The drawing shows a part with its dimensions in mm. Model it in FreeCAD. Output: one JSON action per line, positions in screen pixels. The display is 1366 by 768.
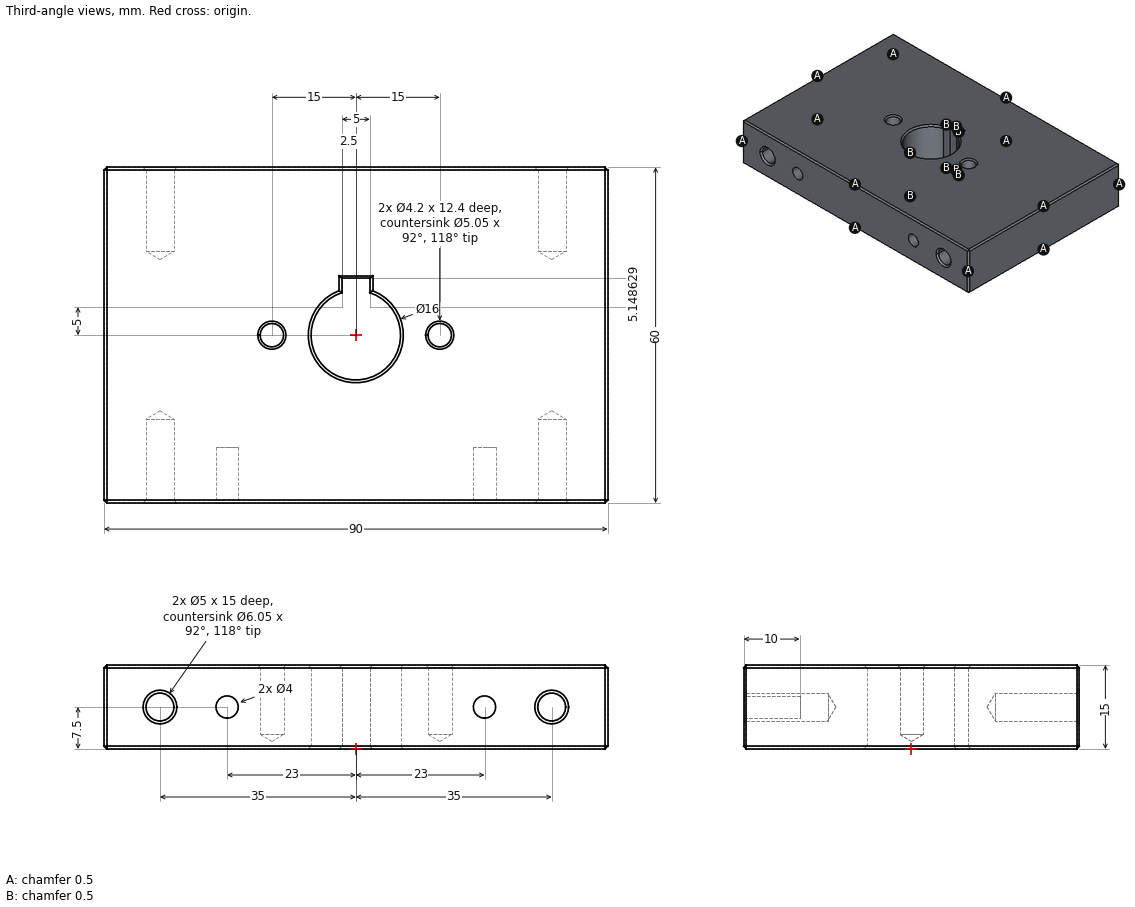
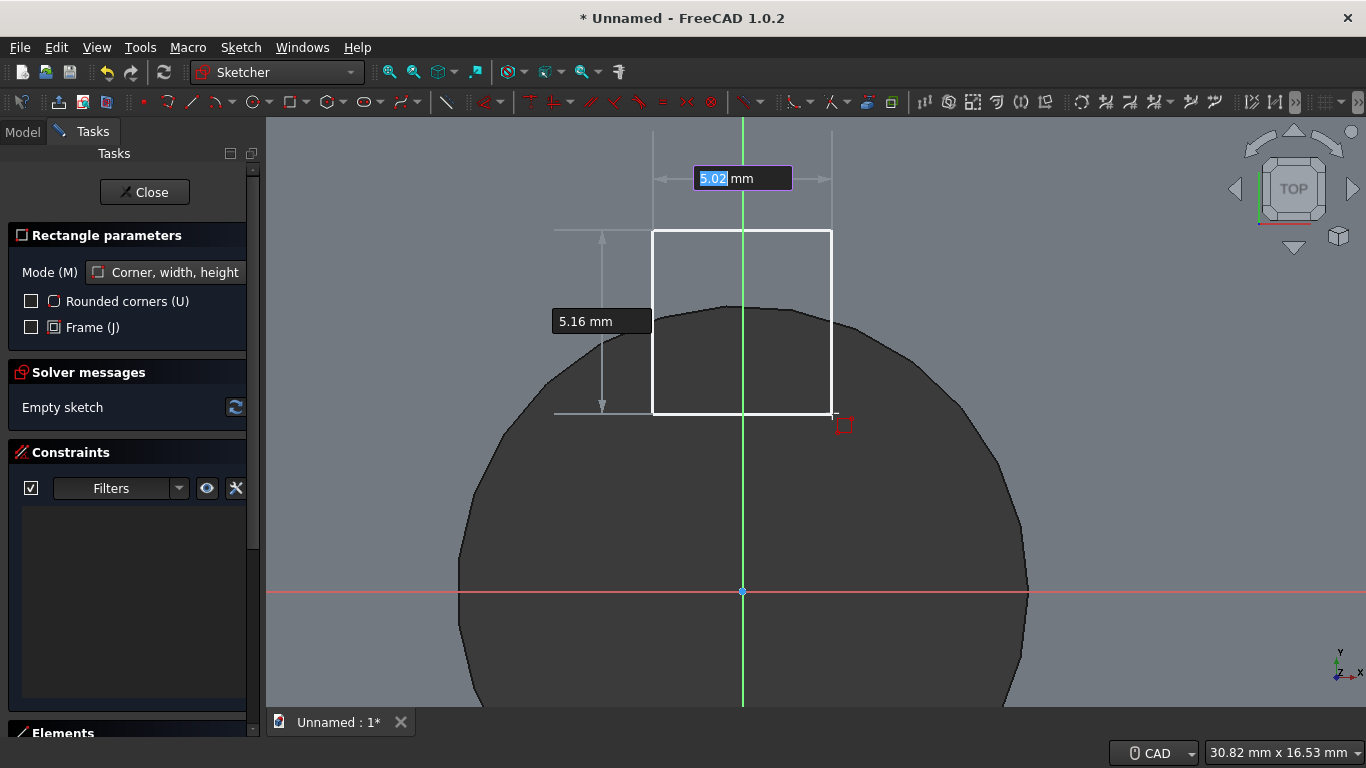
{"action": "type", "text": "5"}
{"action": "key", "text": "Tab"}
{"action": "type", "text": "5.148629"}
{"action": "key", "text": "Return"}
{"action": "key", "text": "Escape"}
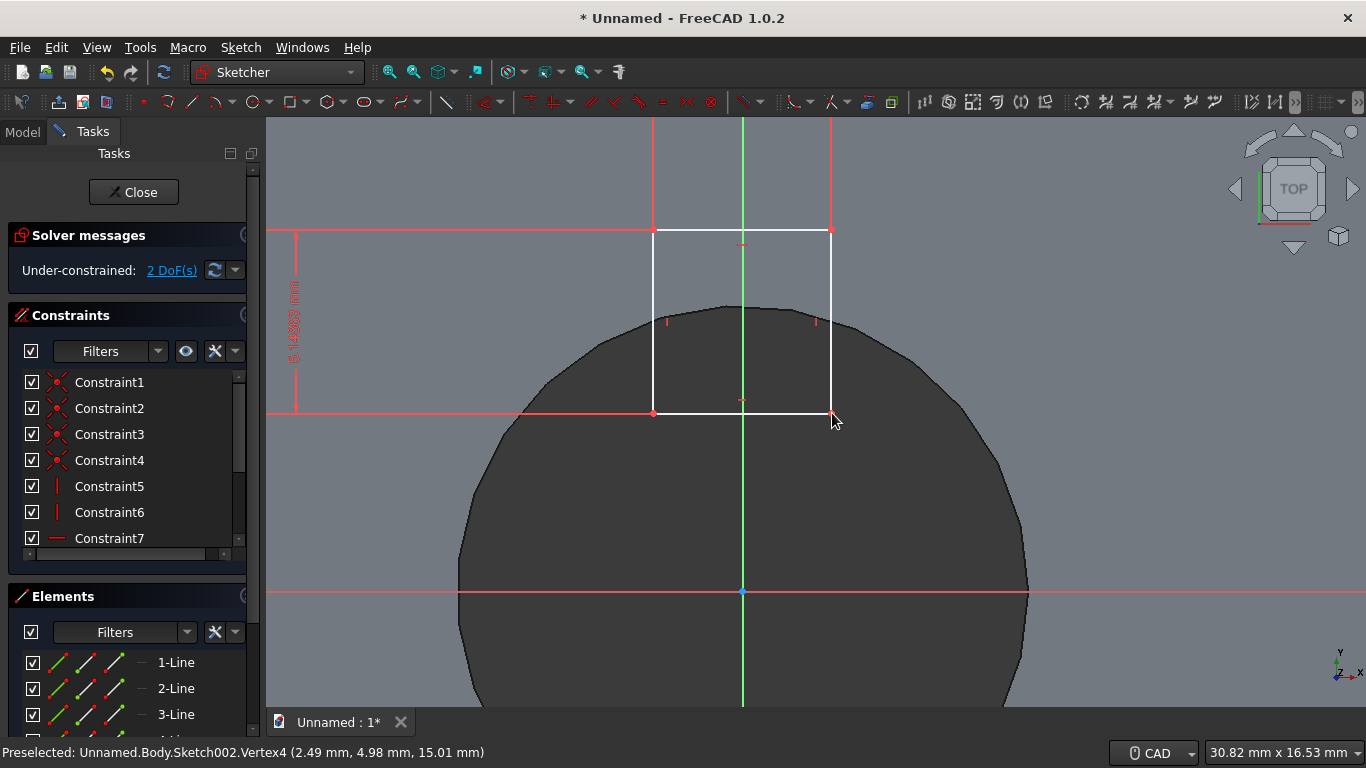
{"action": "key", "text": "d"}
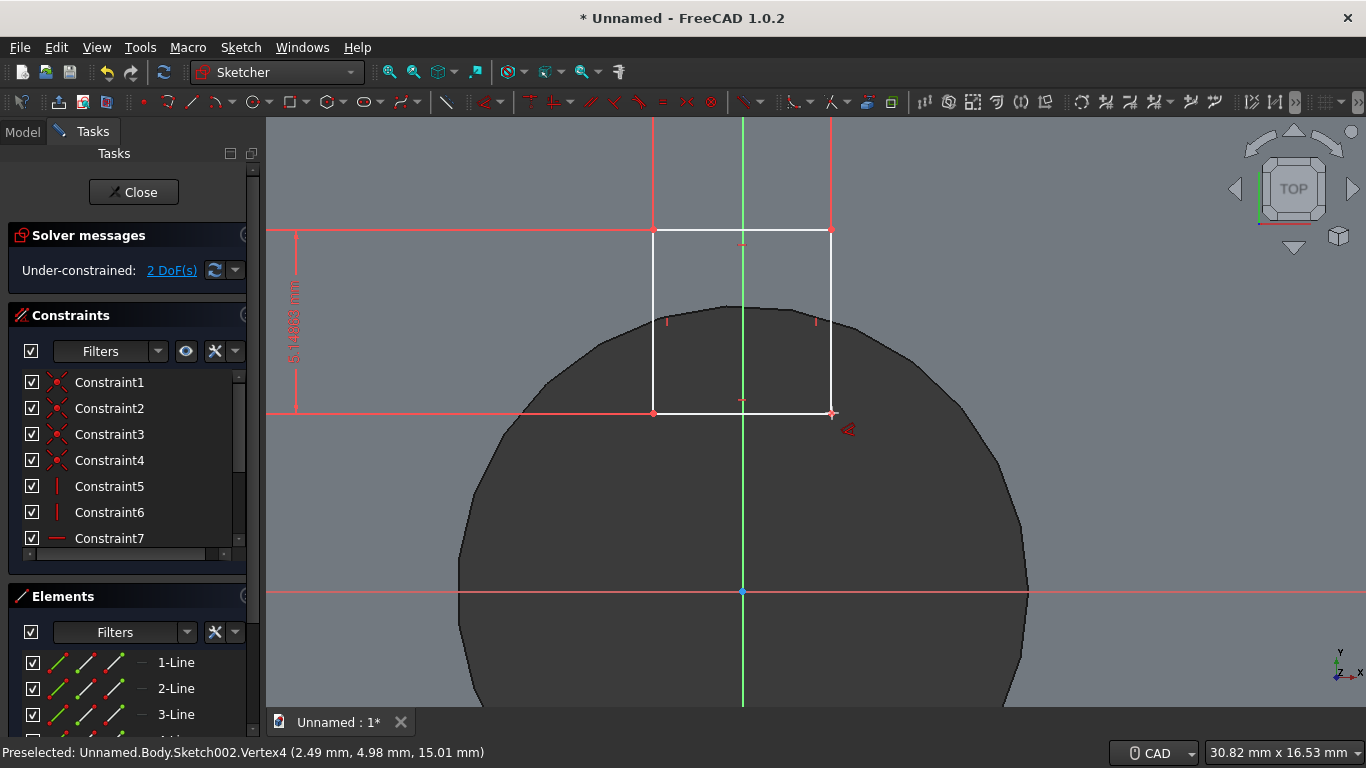
{"action": "left_click", "coordinate": [653, 414]}
{"action": "left_click", "coordinate": [619, 503]}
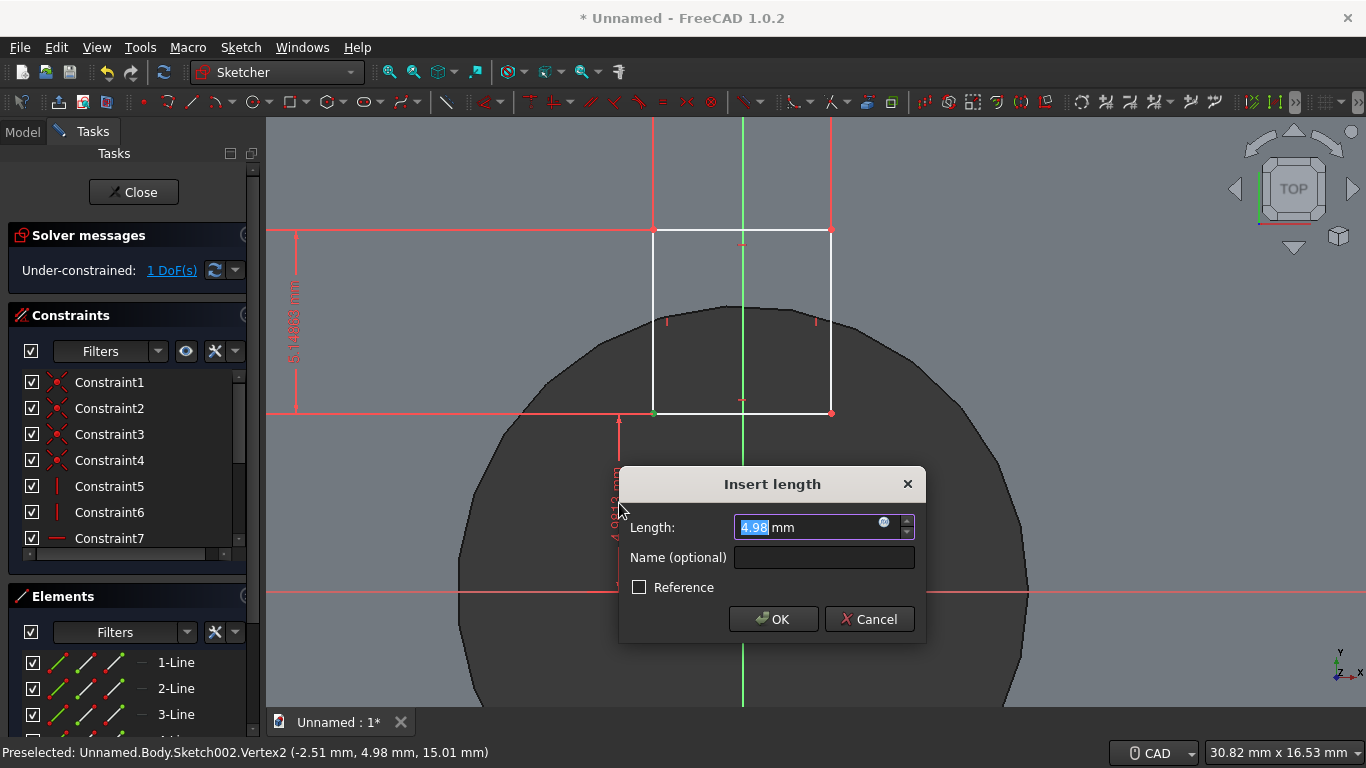
{"action": "type", "text": "5"}
{"action": "key", "text": "Return"}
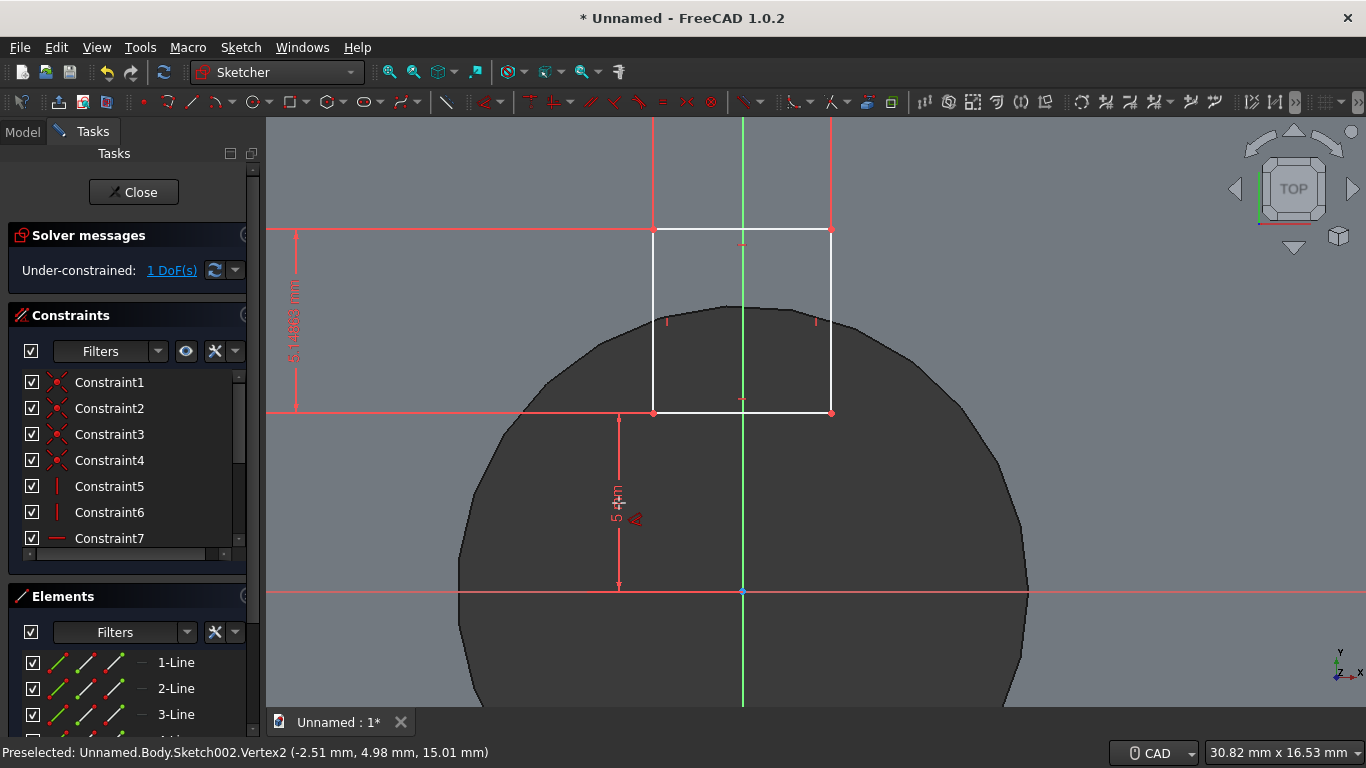
{"action": "left_click", "coordinate": [653, 229]}
{"action": "left_click", "coordinate": [698, 626]}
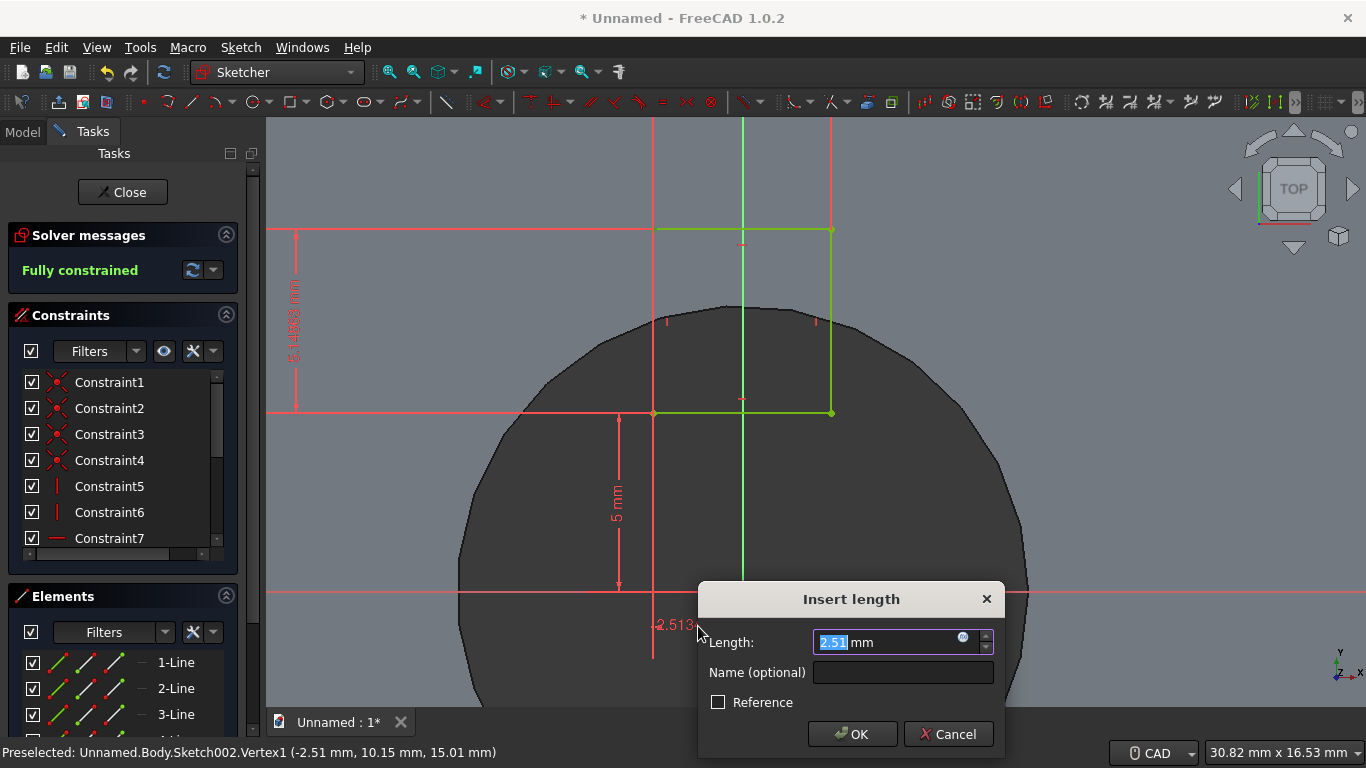
{"action": "type", "text": "2.5"}
{"action": "key", "text": "Return"}
{"action": "key", "text": "Escape"}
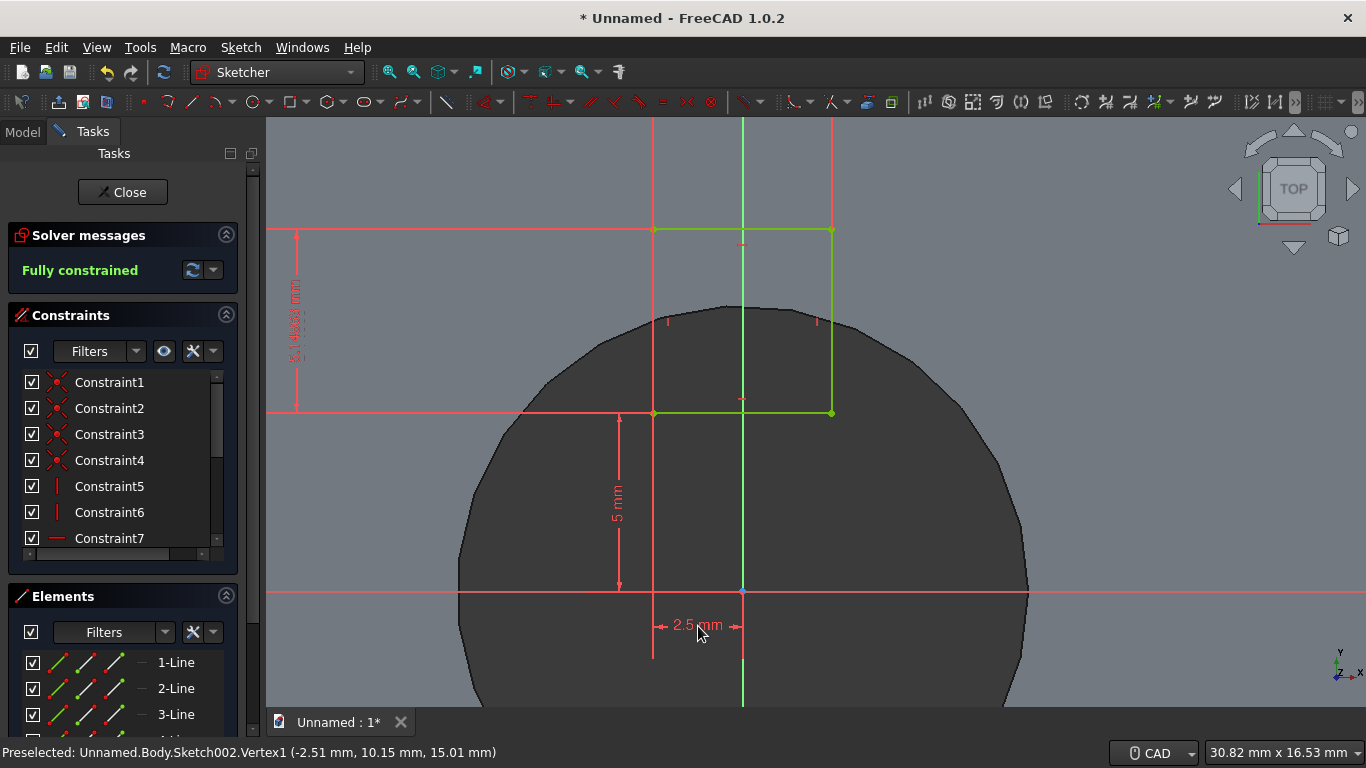
{"action": "left_click", "coordinate": [123, 192]}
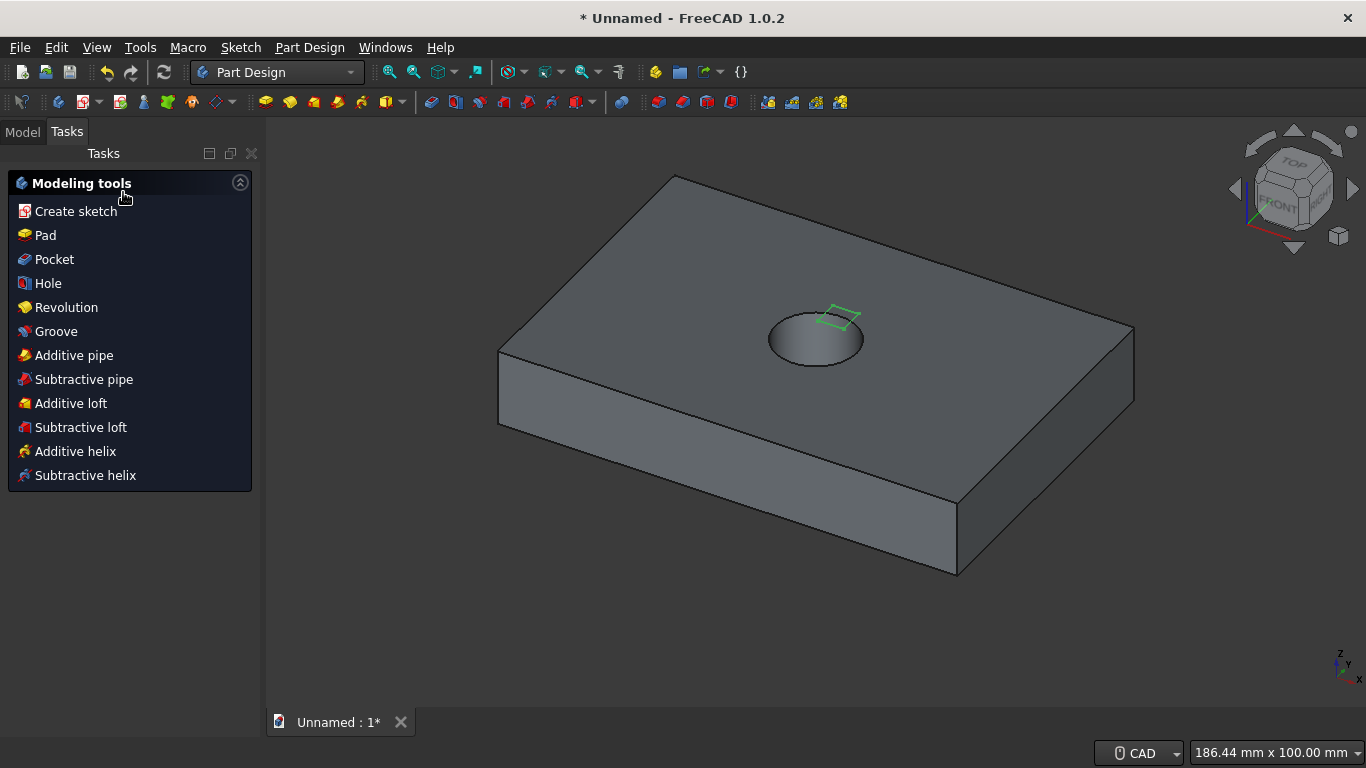
{"action": "left_click", "coordinate": [432, 102]}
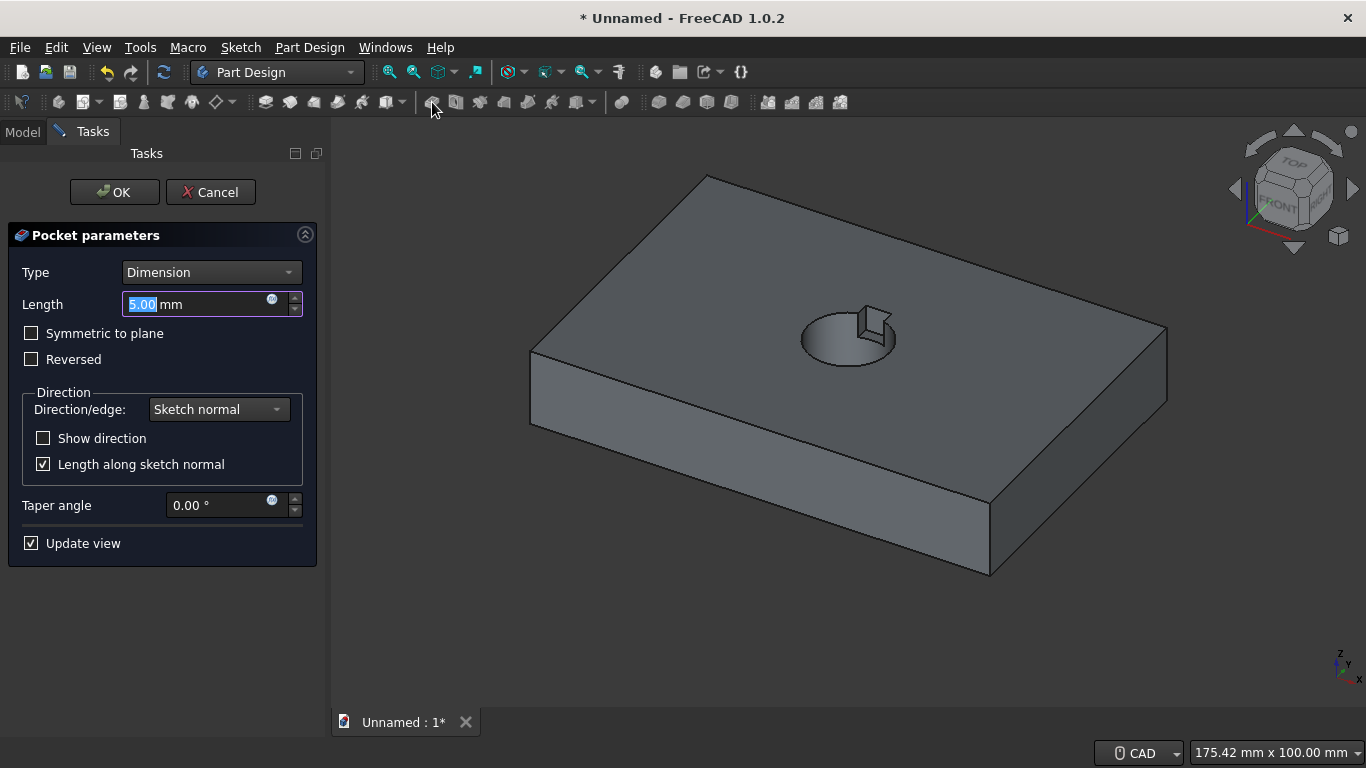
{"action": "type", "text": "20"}
{"action": "key", "text": "Tab"}